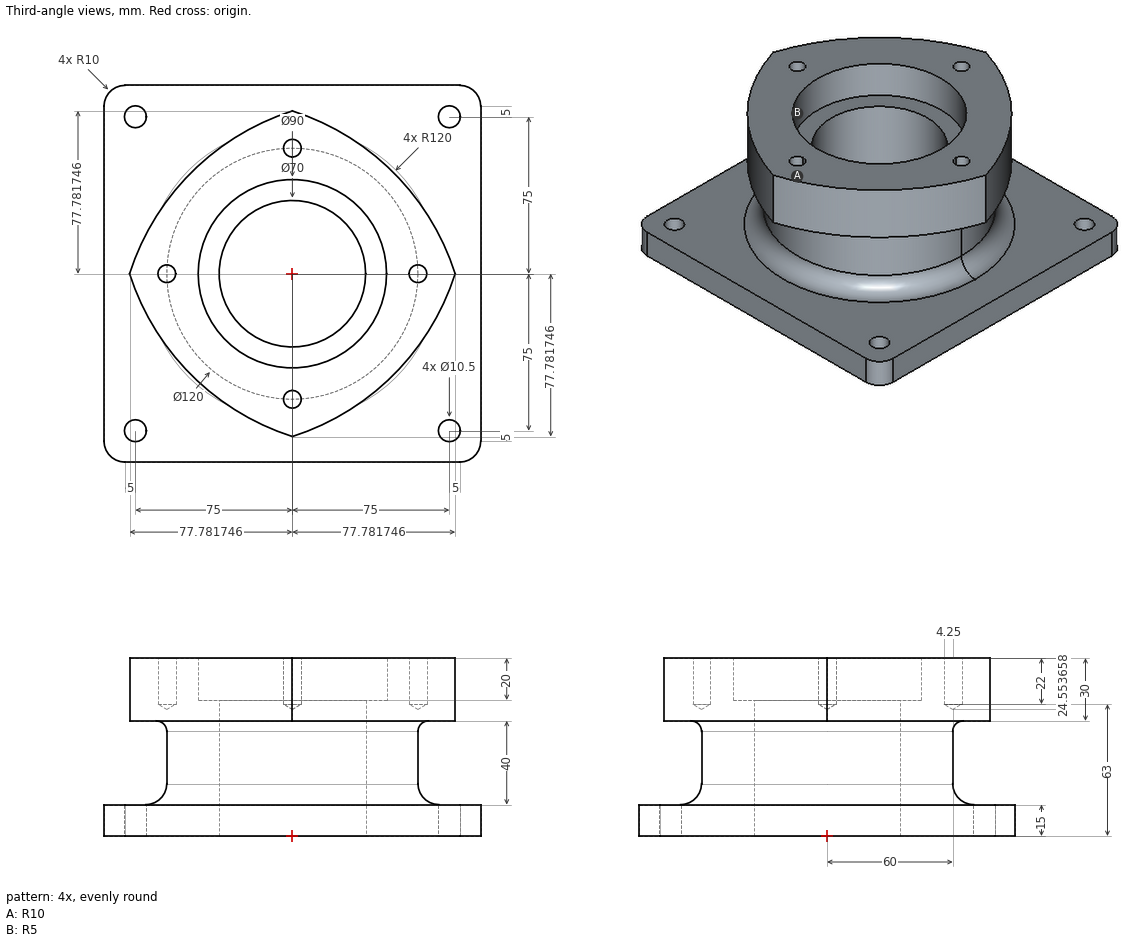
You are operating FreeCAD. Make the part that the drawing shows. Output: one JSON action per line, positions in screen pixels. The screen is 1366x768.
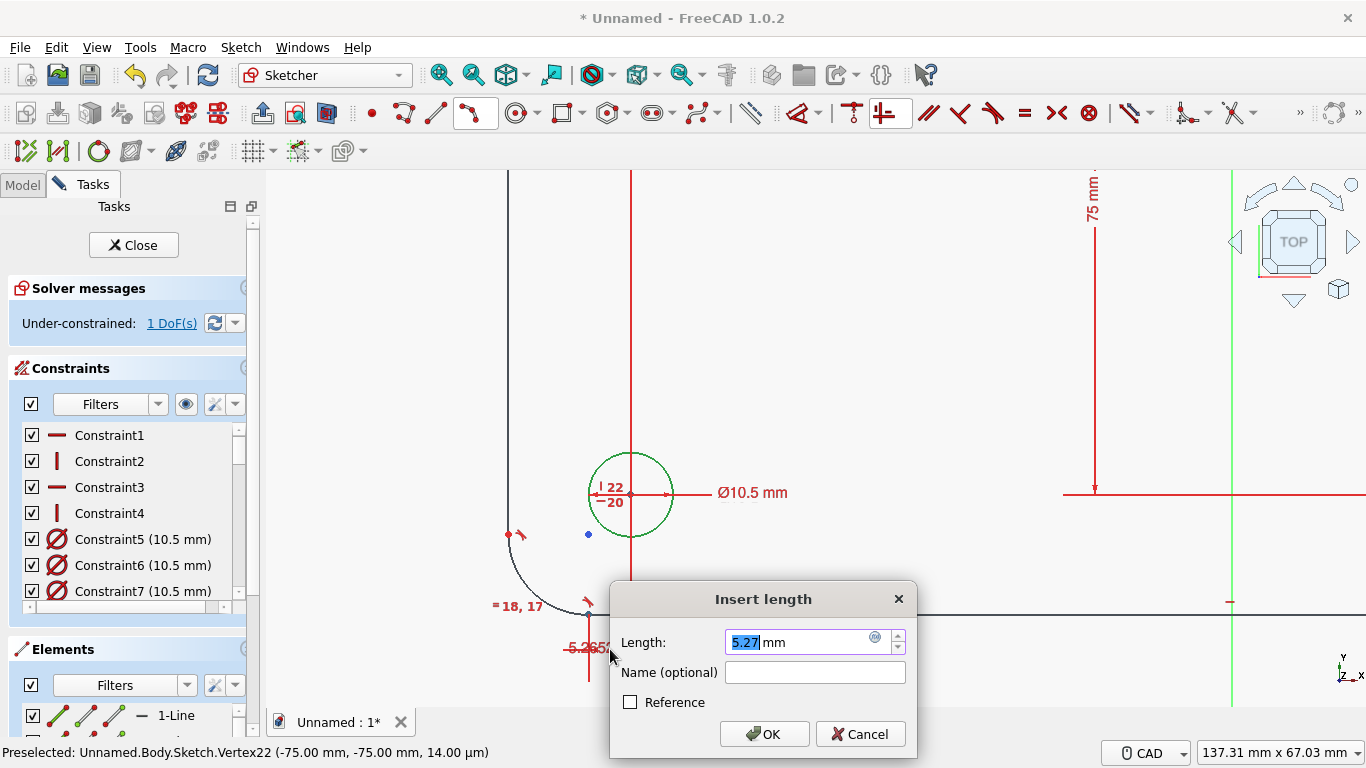
{"action": "type", "text": "5"}
{"action": "key", "text": "Return"}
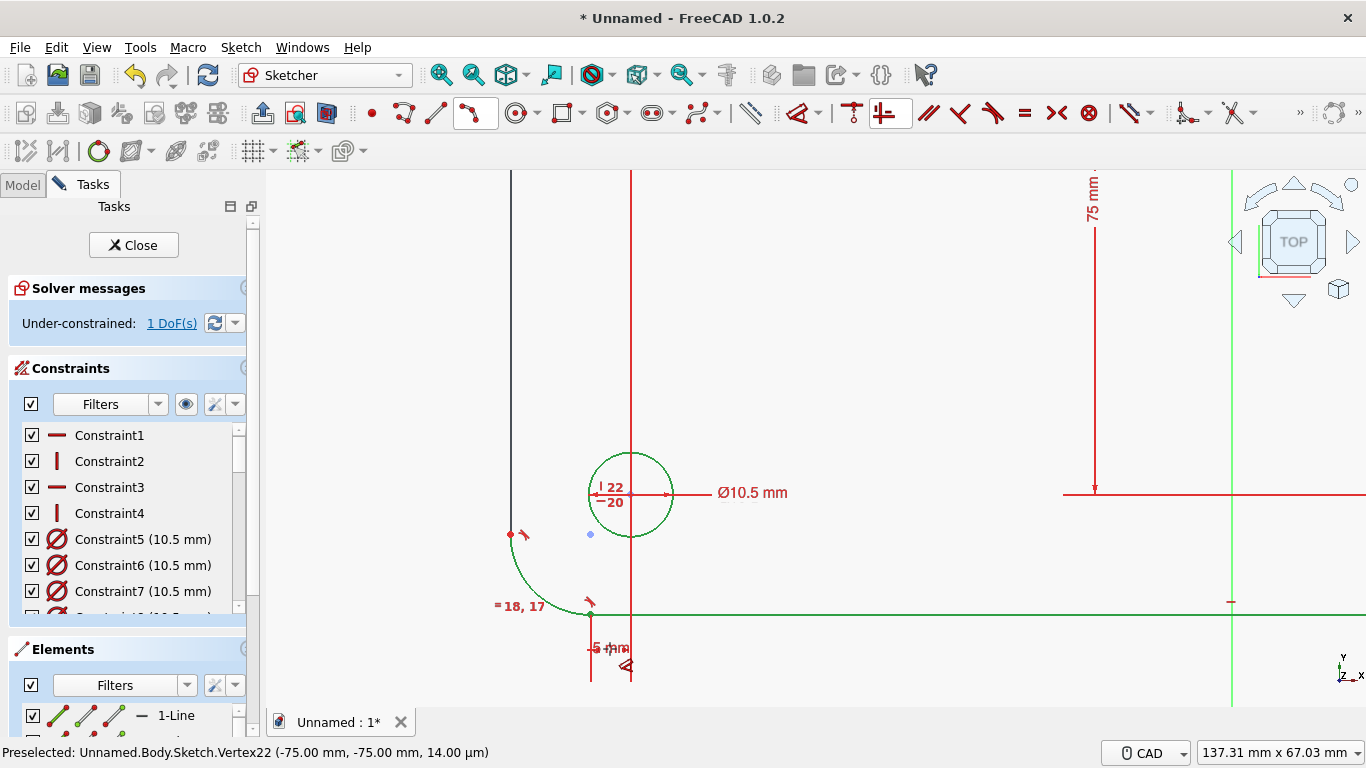
{"action": "scroll", "coordinate": [589, 617], "scroll_direction": "down", "scroll_amount": 7}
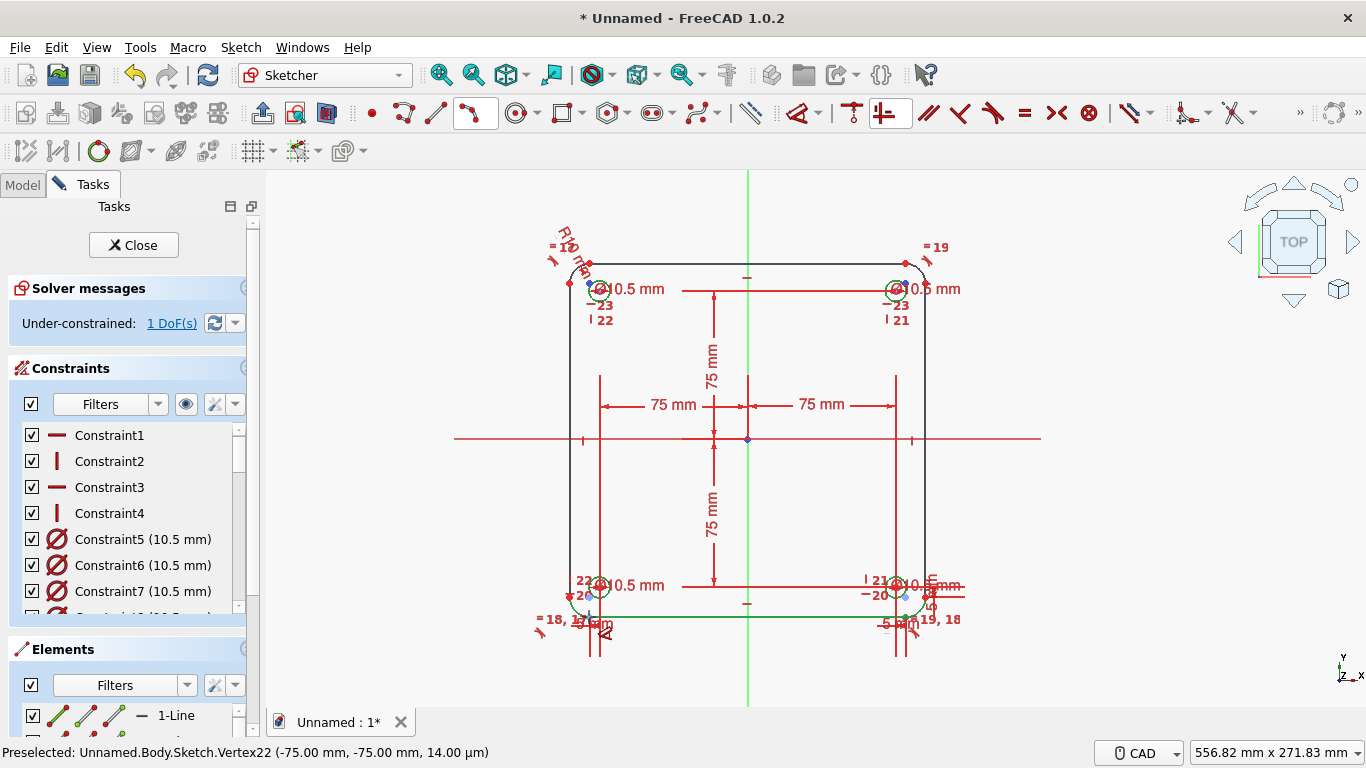
{"action": "scroll", "coordinate": [925, 284], "scroll_direction": "up", "scroll_amount": 7}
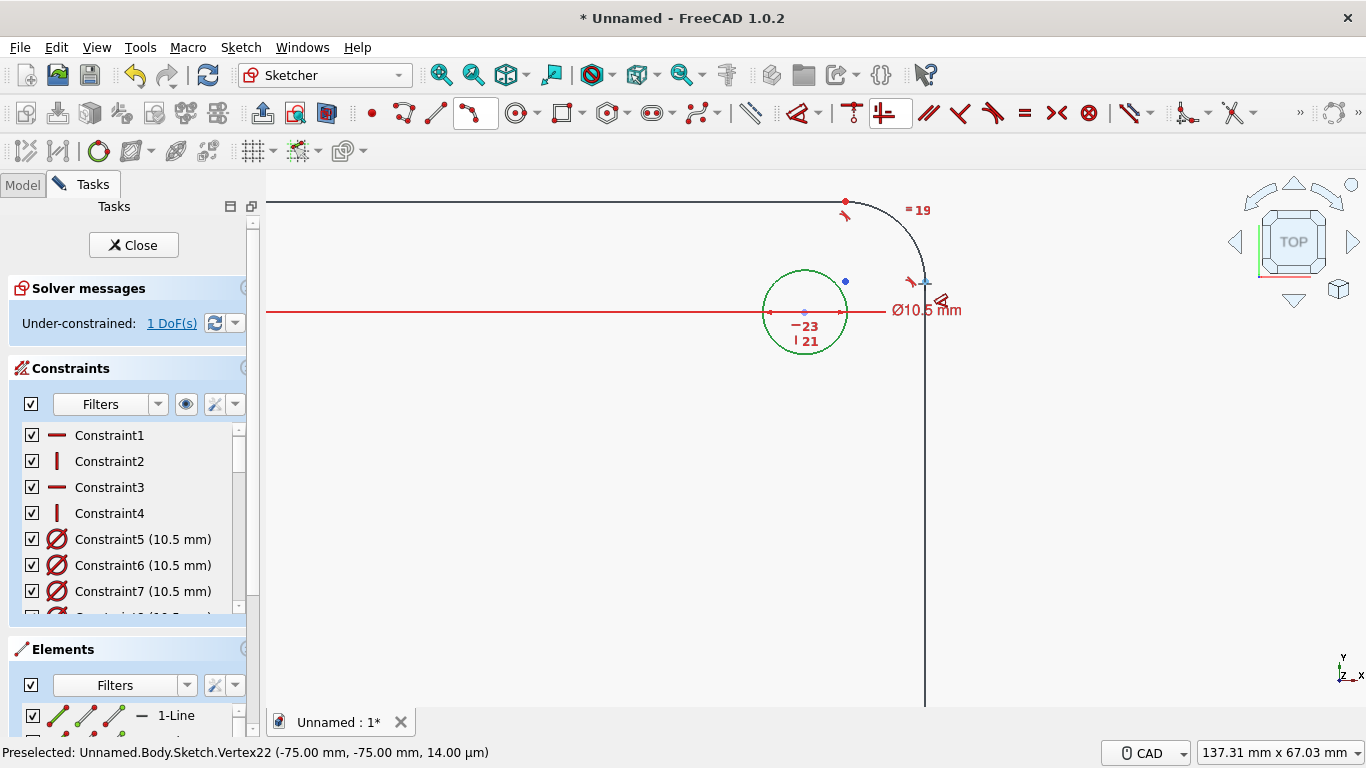
{"action": "left_click", "coordinate": [925, 282]}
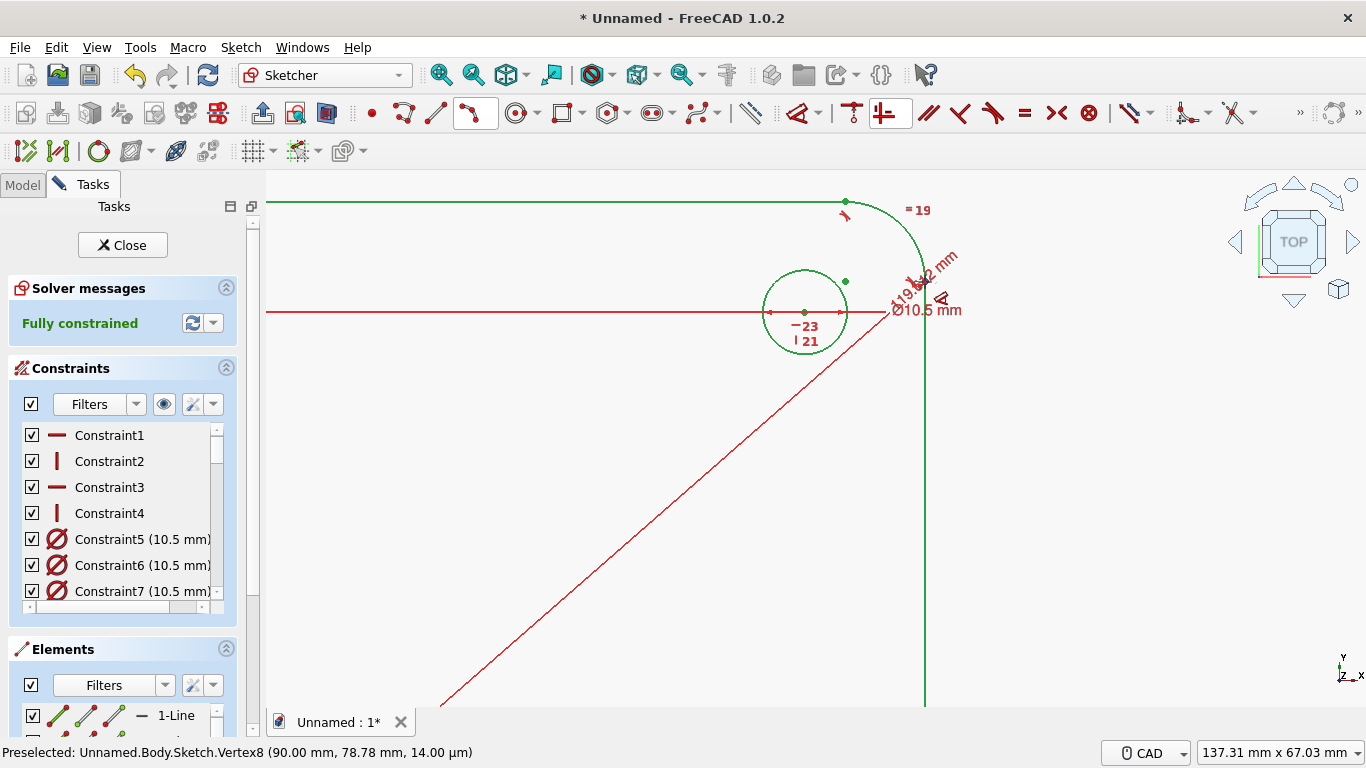
{"action": "left_click", "coordinate": [805, 312]}
{"action": "left_click", "coordinate": [959, 297]}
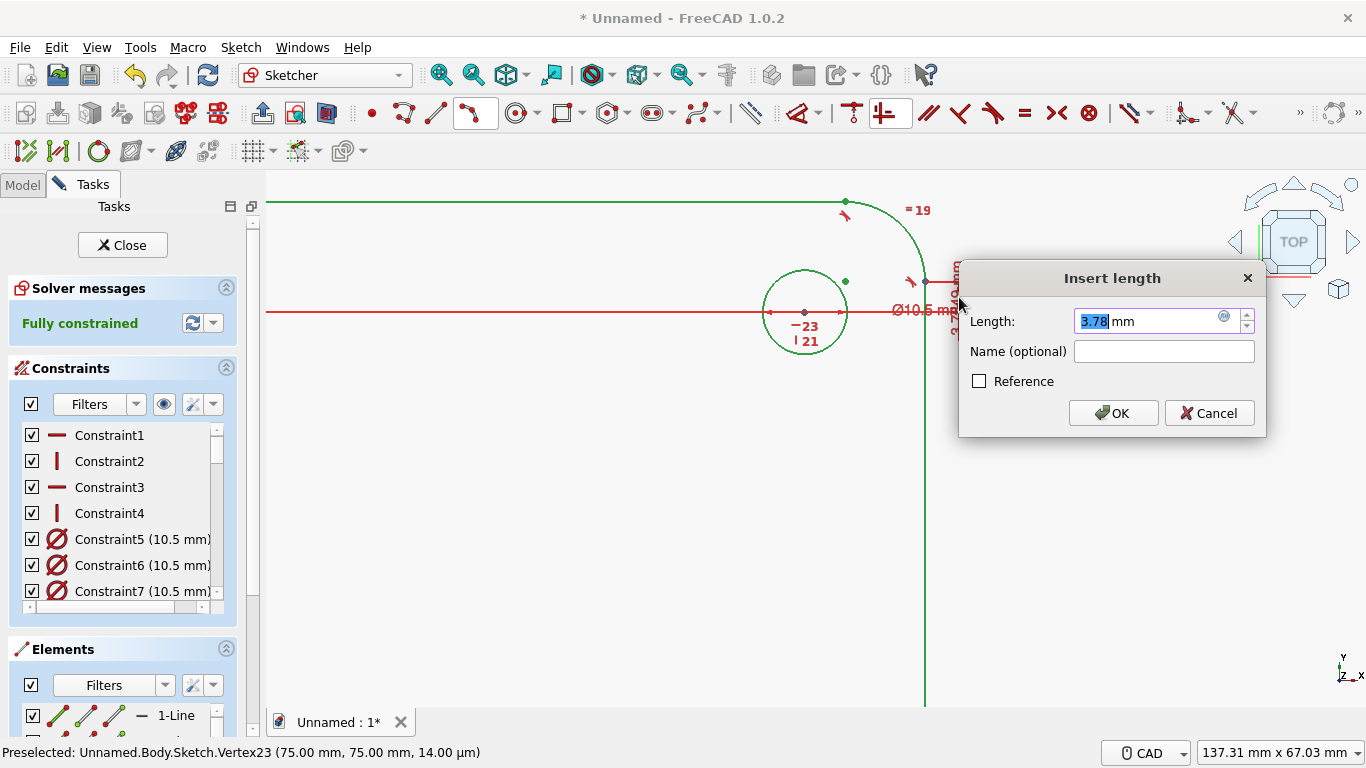
{"action": "type", "text": "5"}
{"action": "key", "text": "Return"}
{"action": "key", "text": "Escape"}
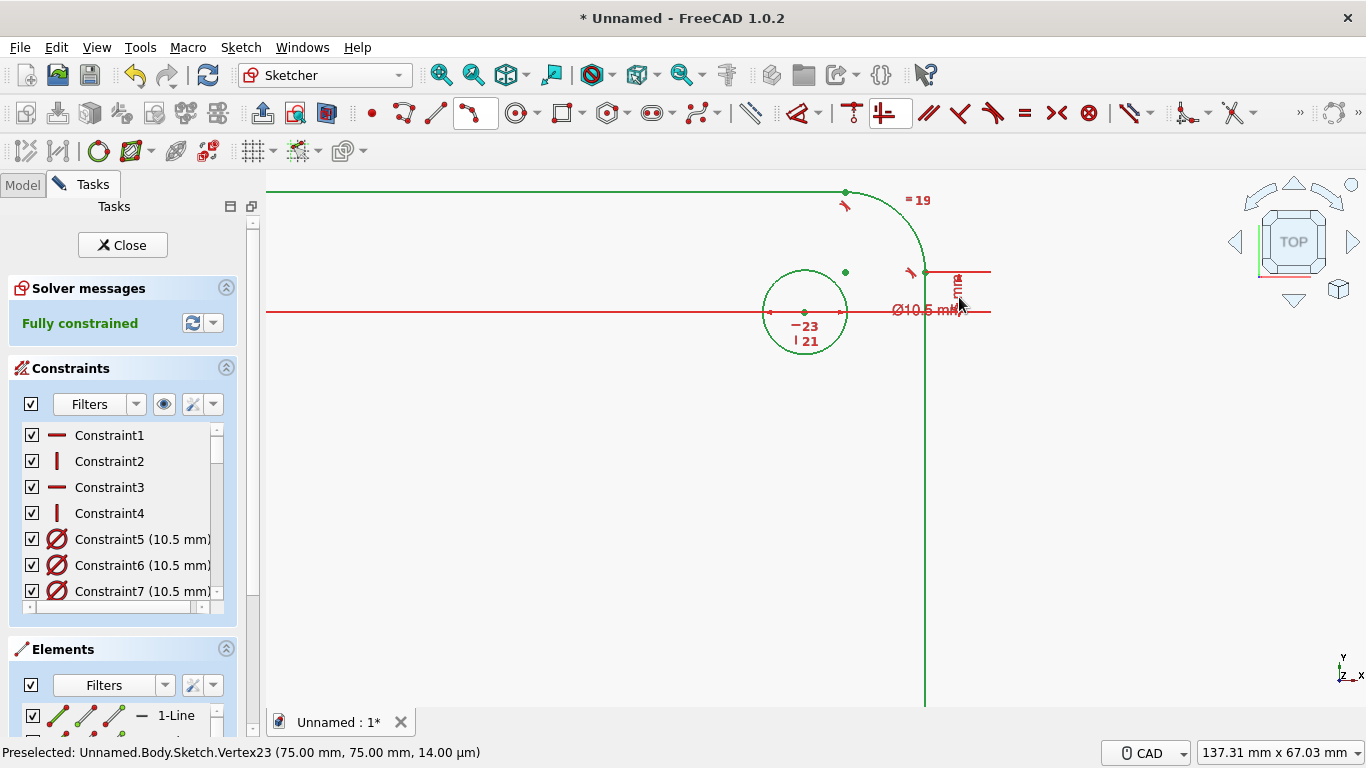
{"action": "left_click", "coordinate": [123, 245]}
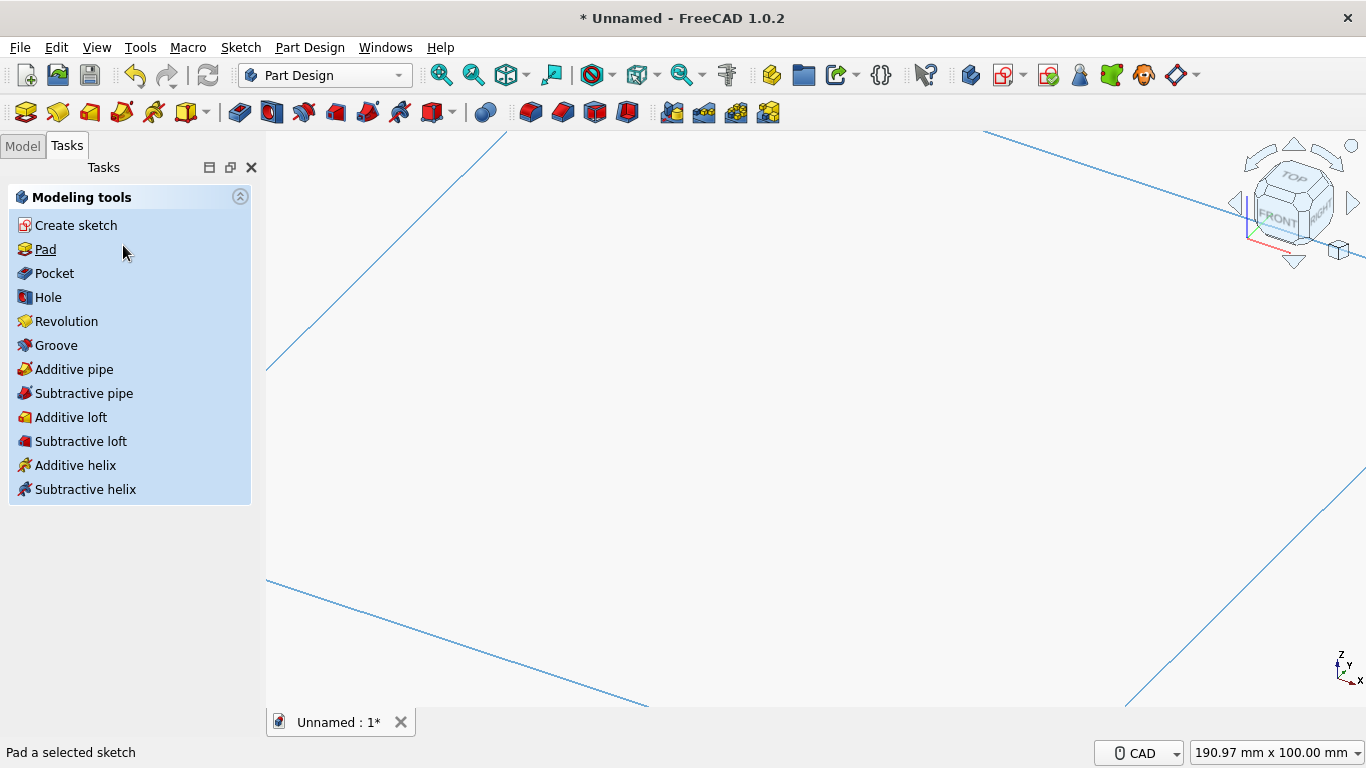
{"action": "left_click", "coordinate": [26, 112]}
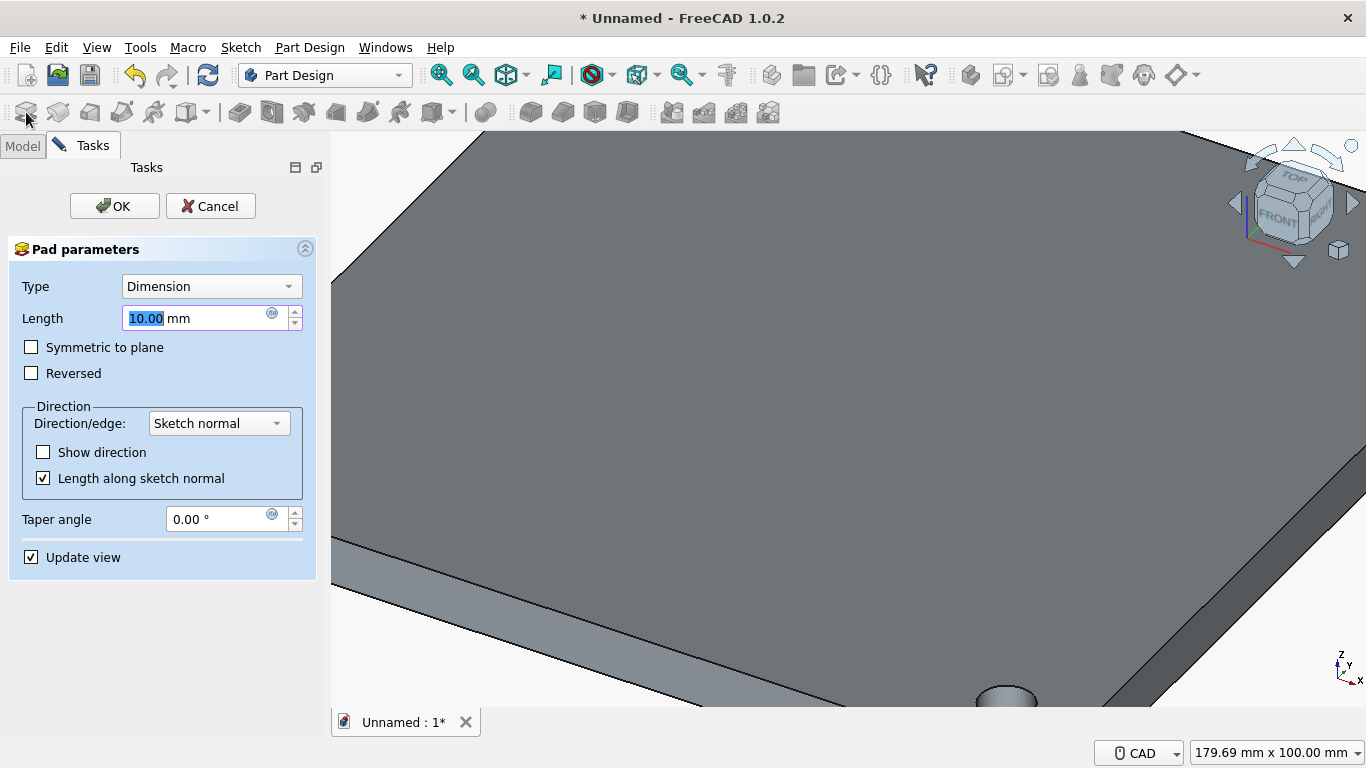
{"action": "type", "text": "15"}
{"action": "key", "text": "Tab"}